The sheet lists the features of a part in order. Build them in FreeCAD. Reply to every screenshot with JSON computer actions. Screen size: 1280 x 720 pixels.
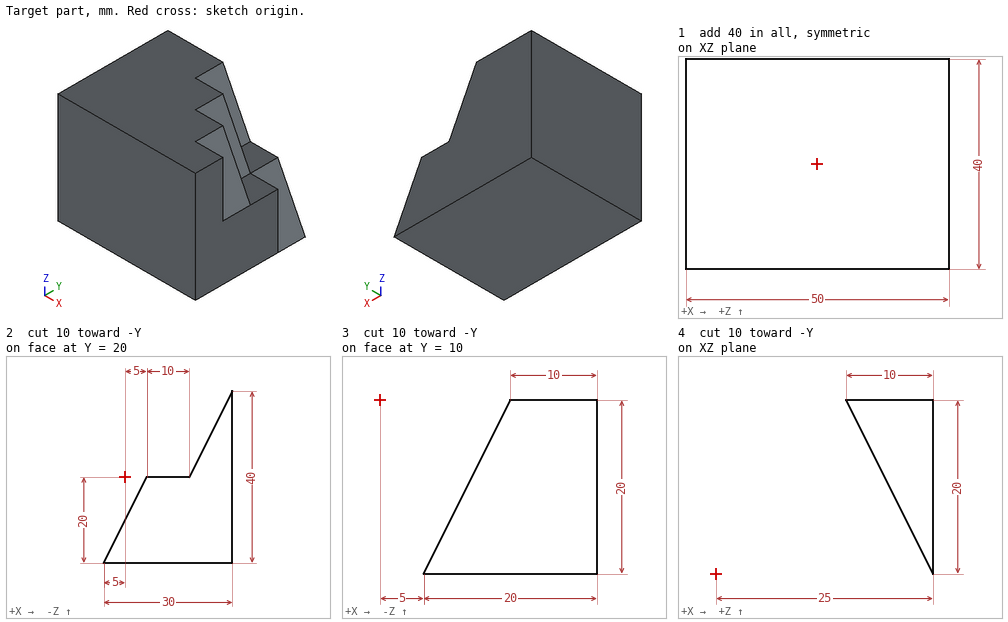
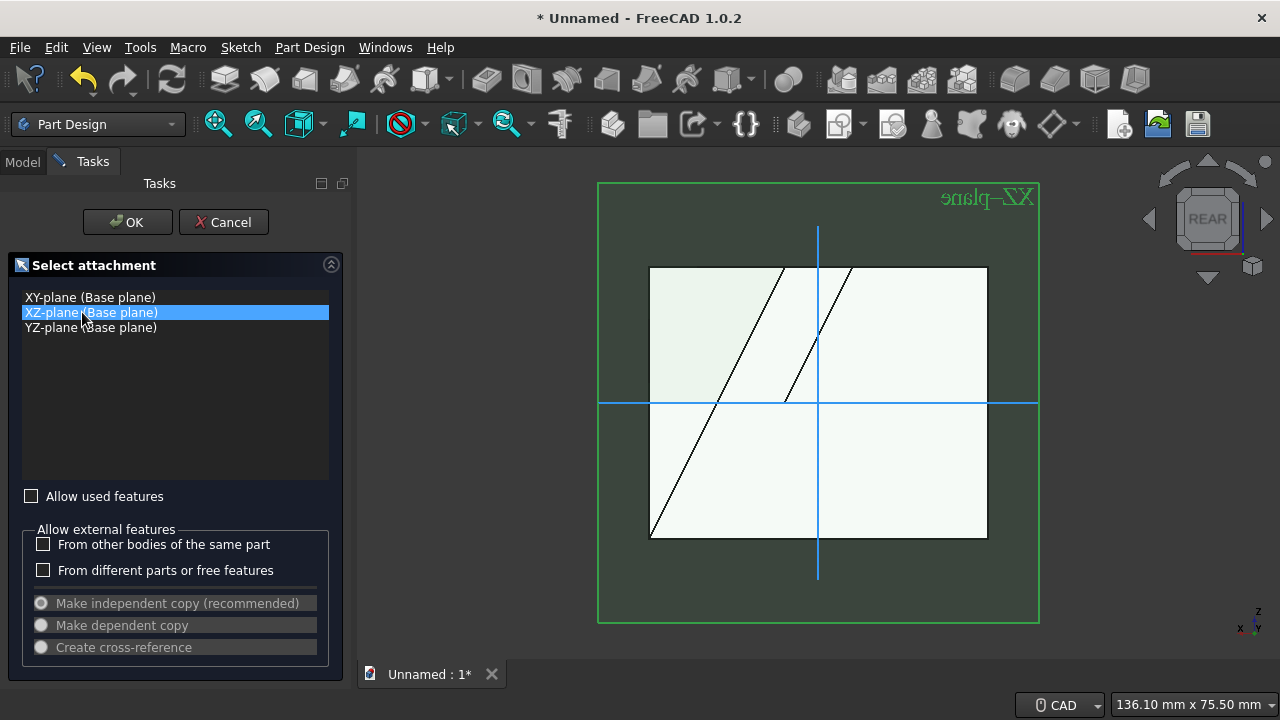
{"action": "left_click", "coordinate": [128, 222]}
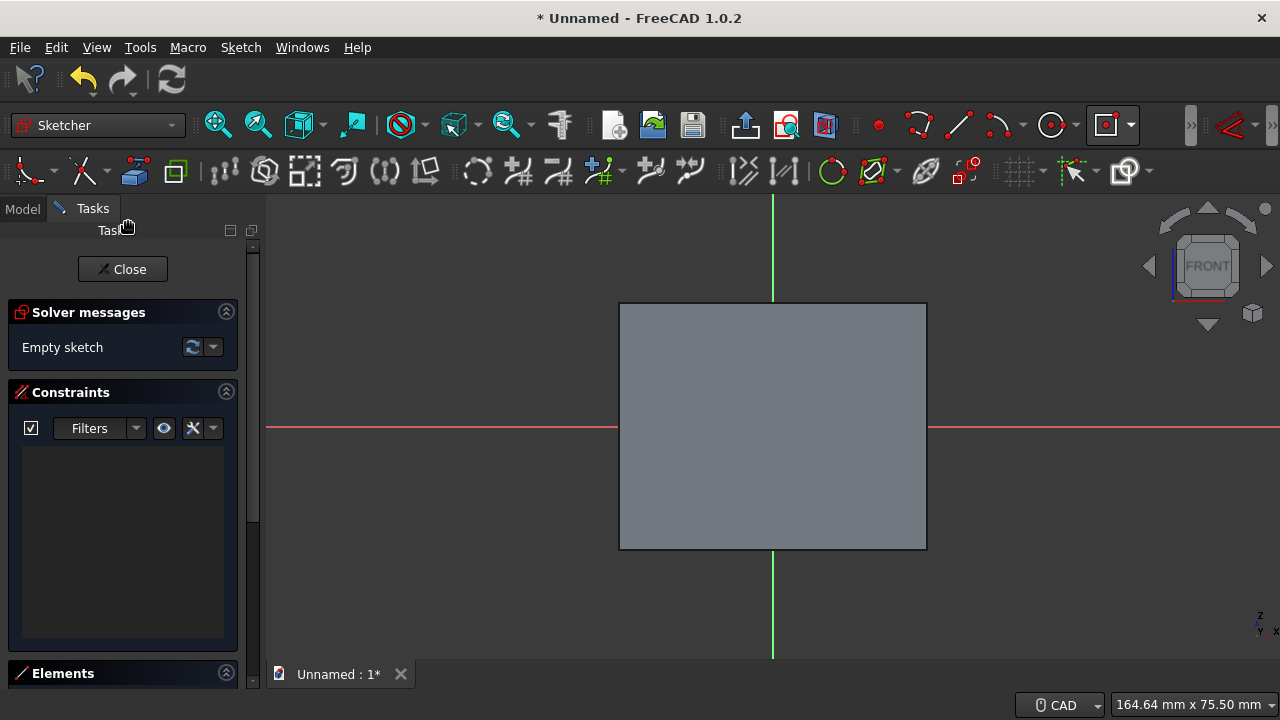
{"action": "left_click", "coordinate": [826, 126]}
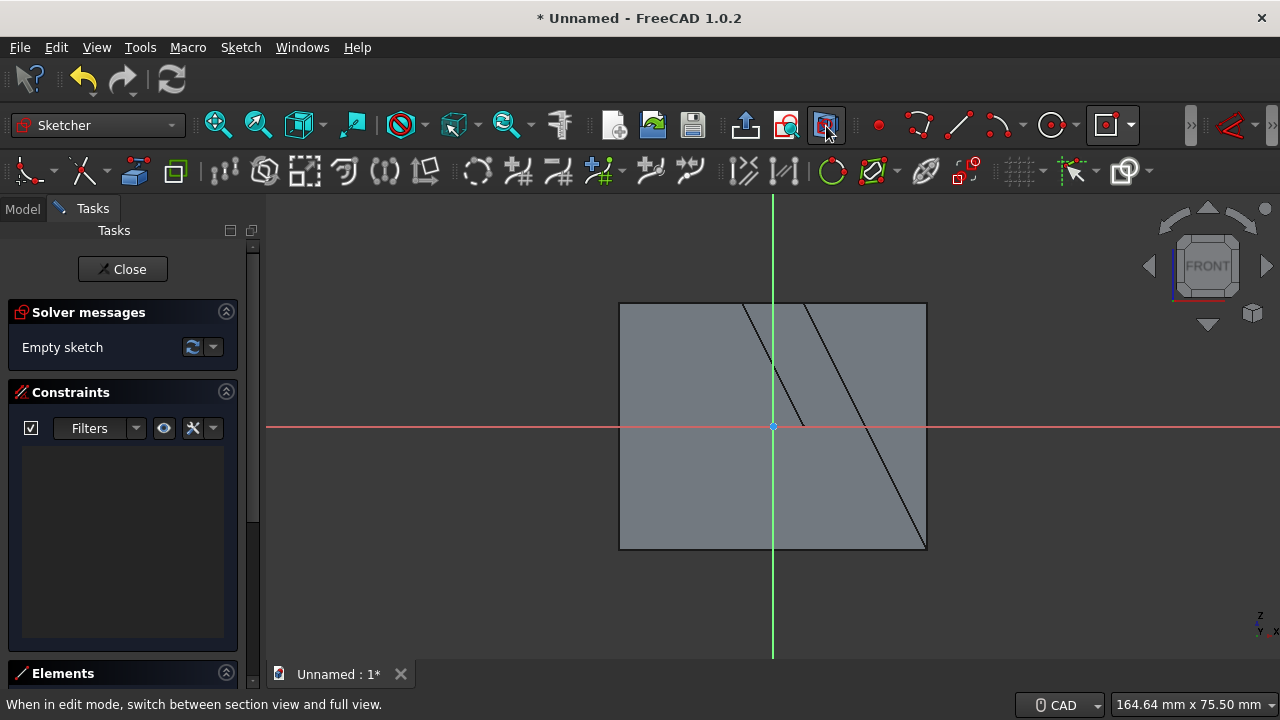
{"action": "scroll", "coordinate": [969, 315], "scroll_direction": "up", "scroll_amount": 4}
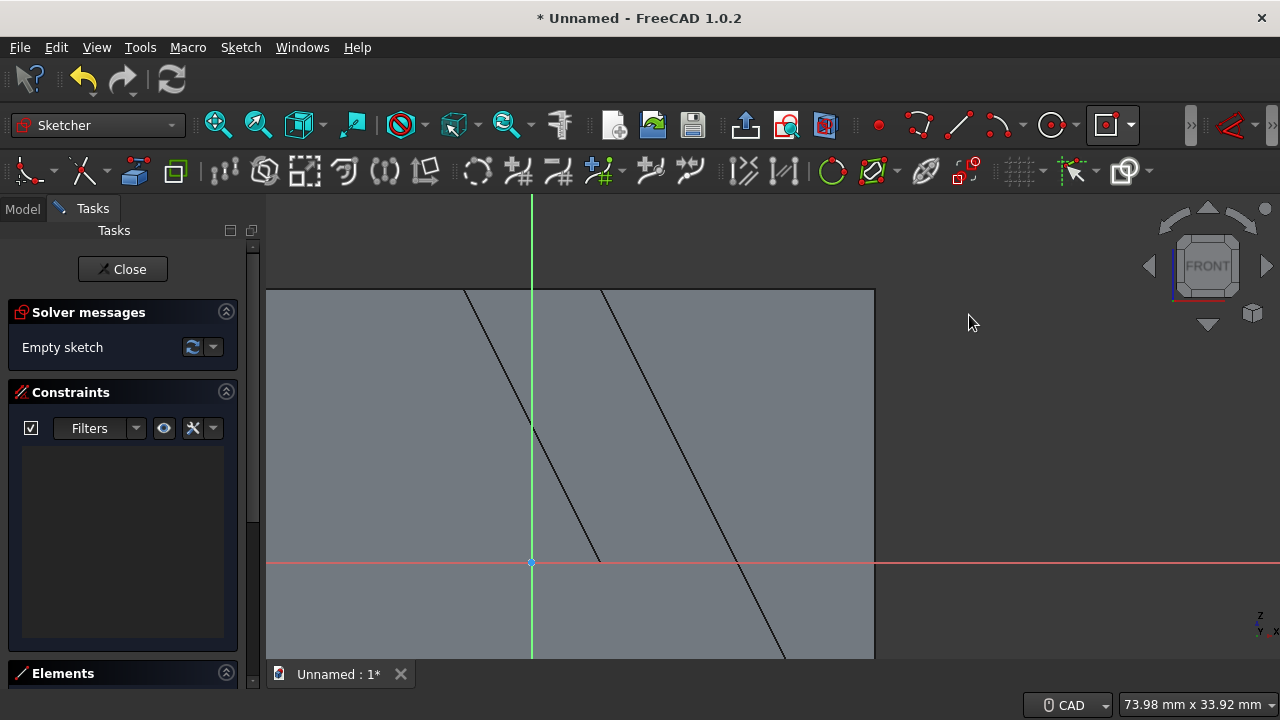
{"action": "left_click", "coordinate": [920, 126]}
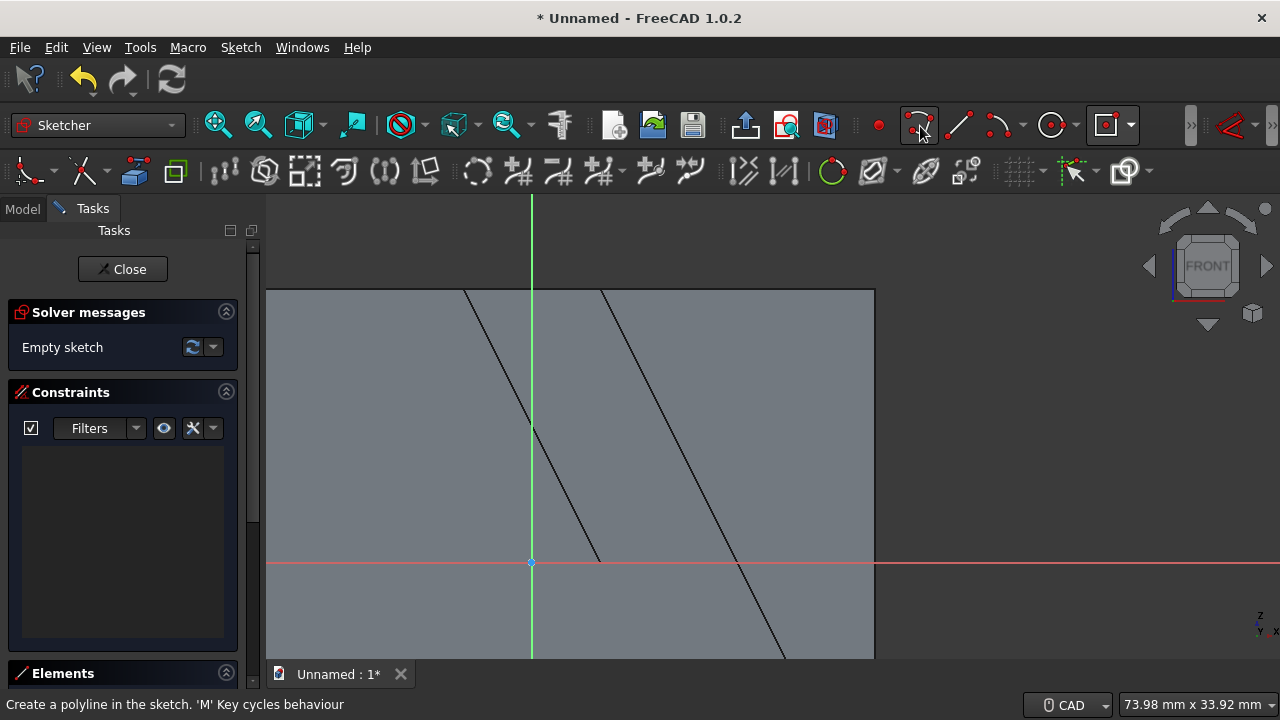
{"action": "left_click", "coordinate": [875, 563]}
{"action": "left_click", "coordinate": [738, 289]}
{"action": "left_click", "coordinate": [875, 289]}
{"action": "left_click", "coordinate": [875, 563]}
{"action": "key", "text": "Escape"}
{"action": "key", "text": "Escape"}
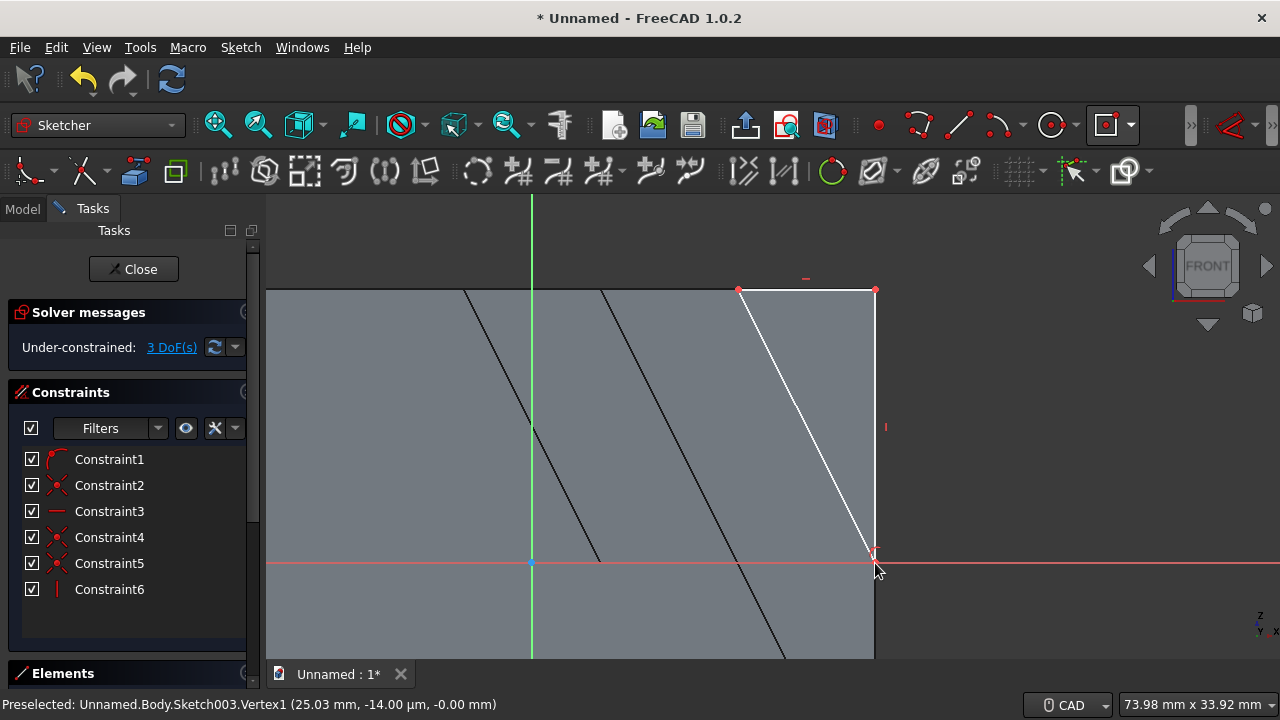
{"action": "left_click", "coordinate": [1230, 126]}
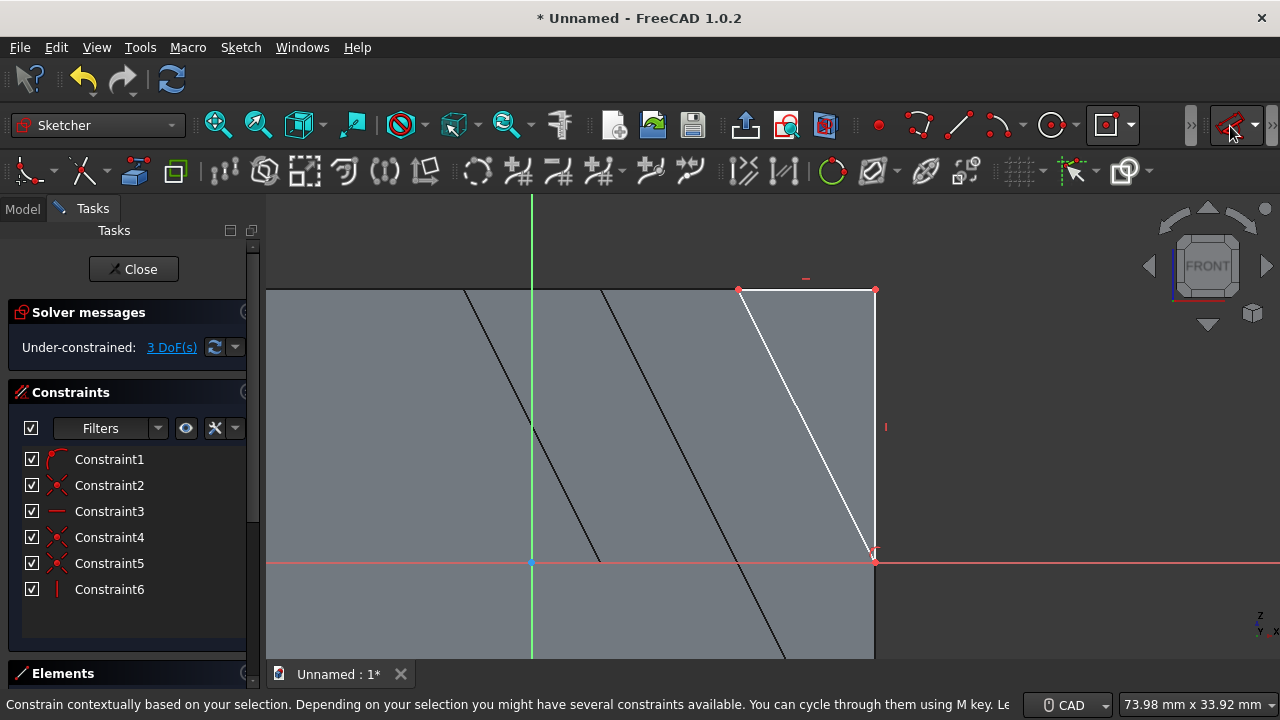
{"action": "left_click", "coordinate": [779, 290]}
{"action": "left_click", "coordinate": [807, 256]}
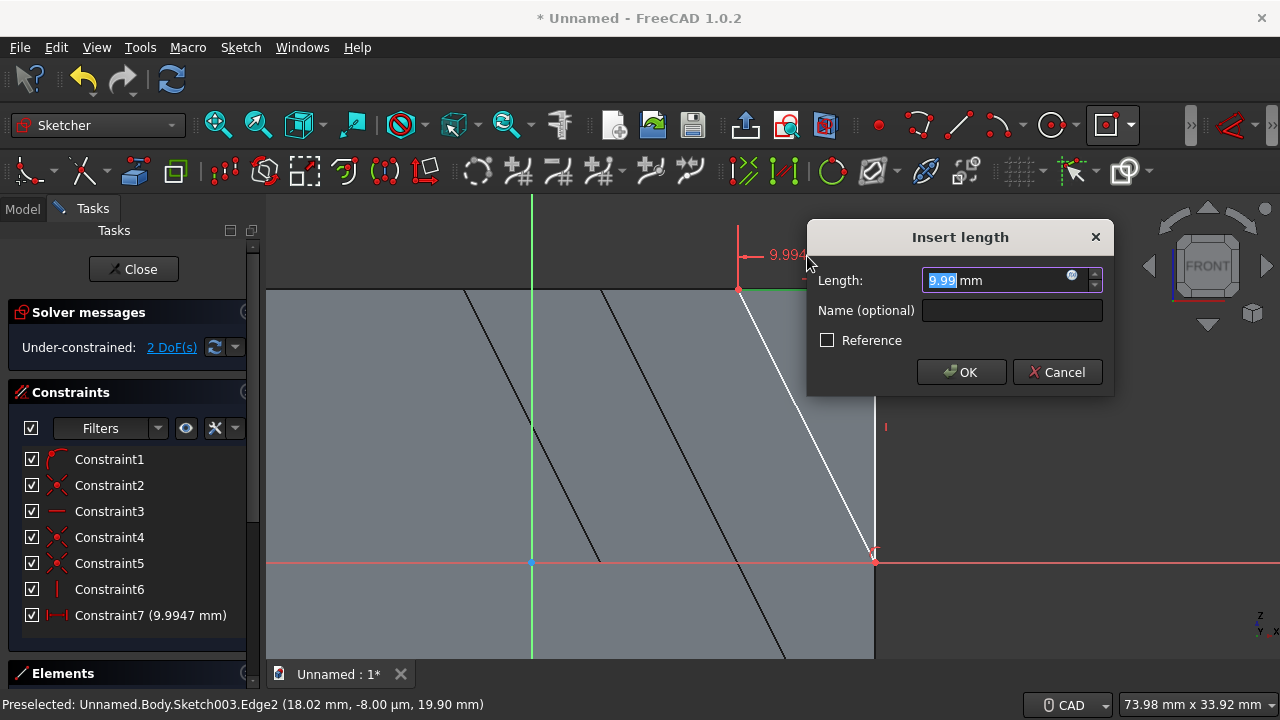
{"action": "type", "text": "10"}
{"action": "key", "text": "Return"}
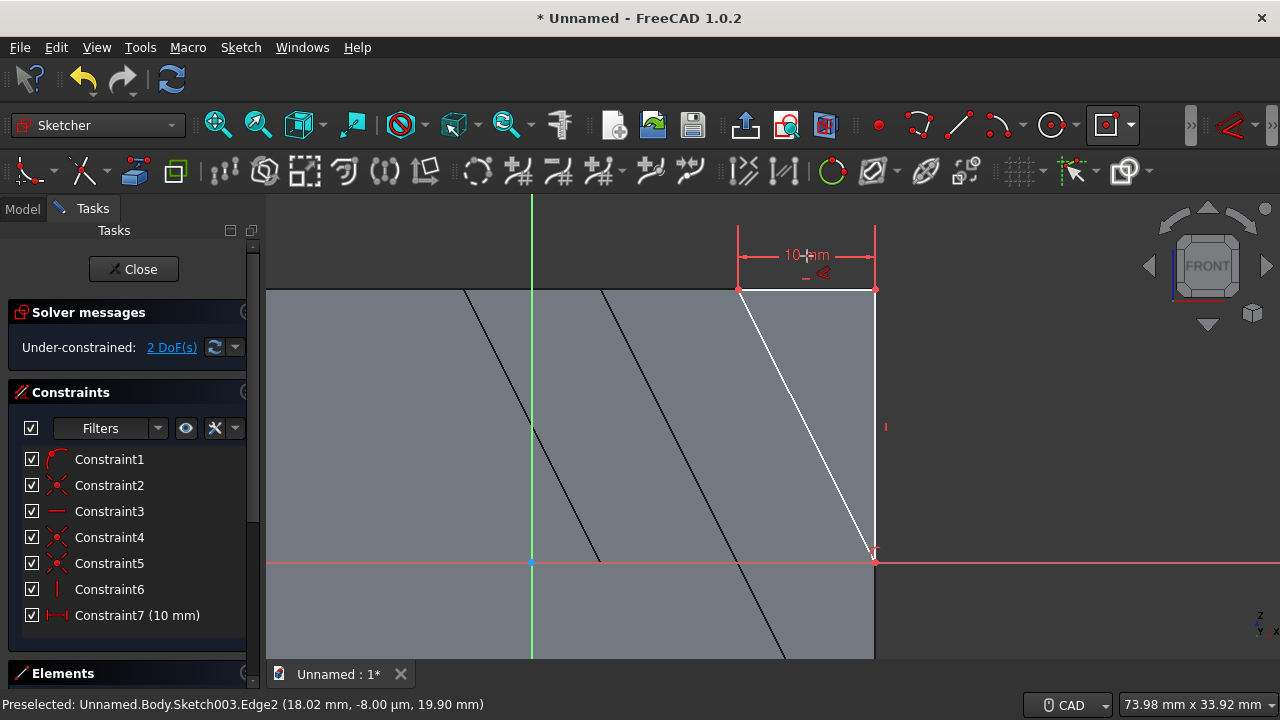
{"action": "left_click", "coordinate": [875, 372]}
{"action": "left_click", "coordinate": [909, 426]}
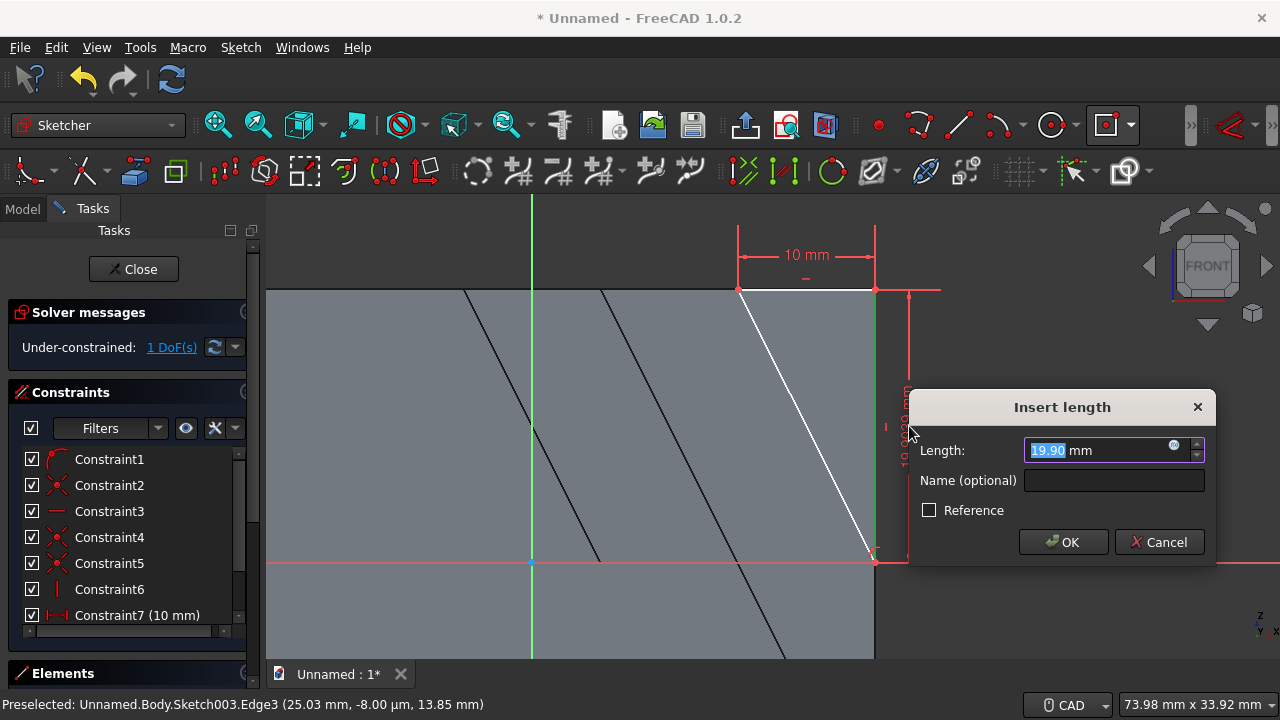
{"action": "type", "text": "20"}
{"action": "key", "text": "Return"}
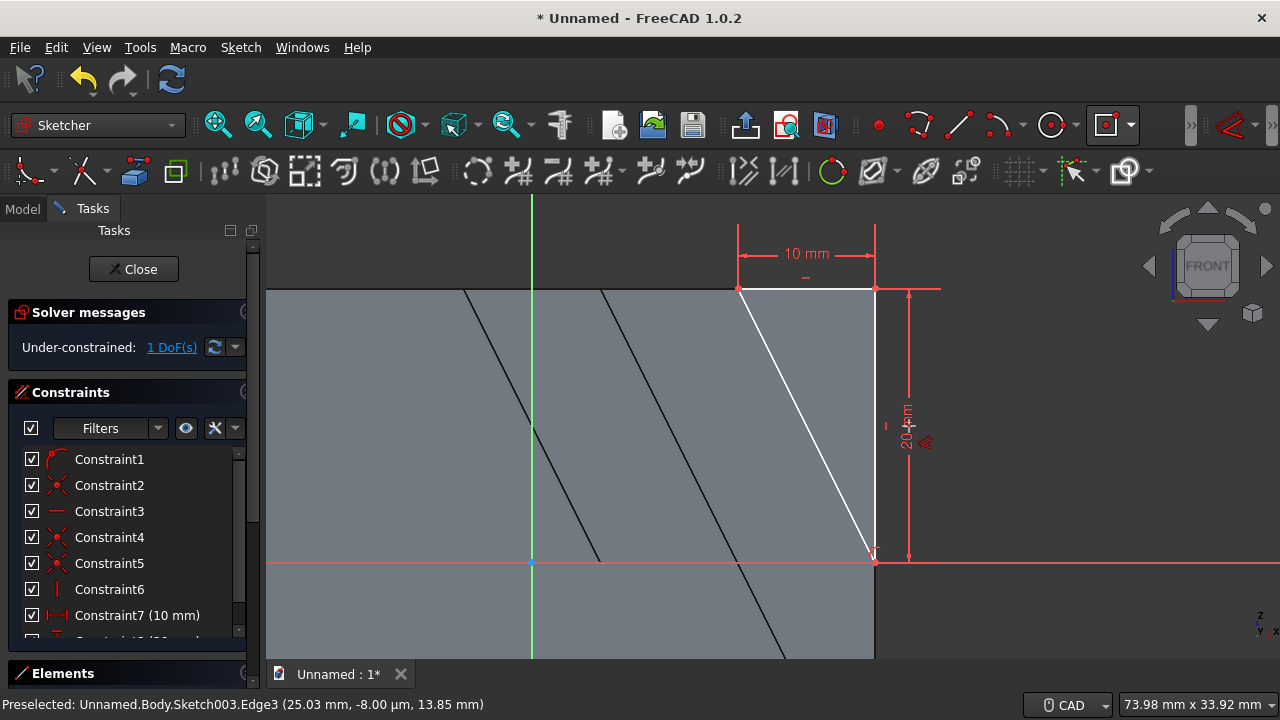
{"action": "left_click", "coordinate": [875, 563]}
{"action": "left_click", "coordinate": [704, 597]}